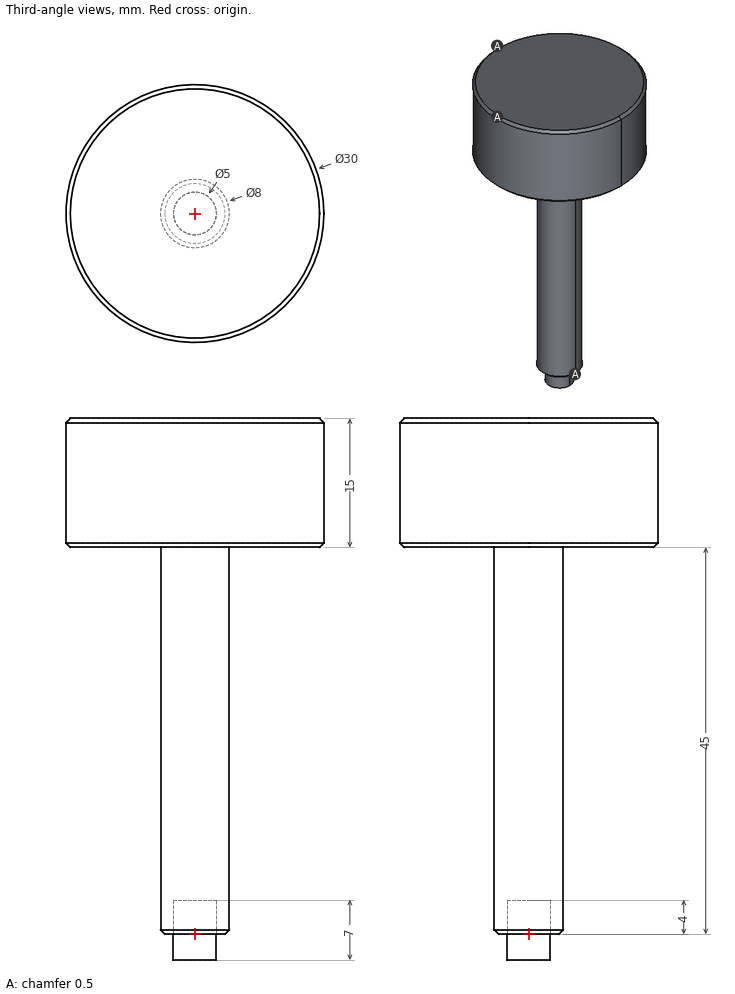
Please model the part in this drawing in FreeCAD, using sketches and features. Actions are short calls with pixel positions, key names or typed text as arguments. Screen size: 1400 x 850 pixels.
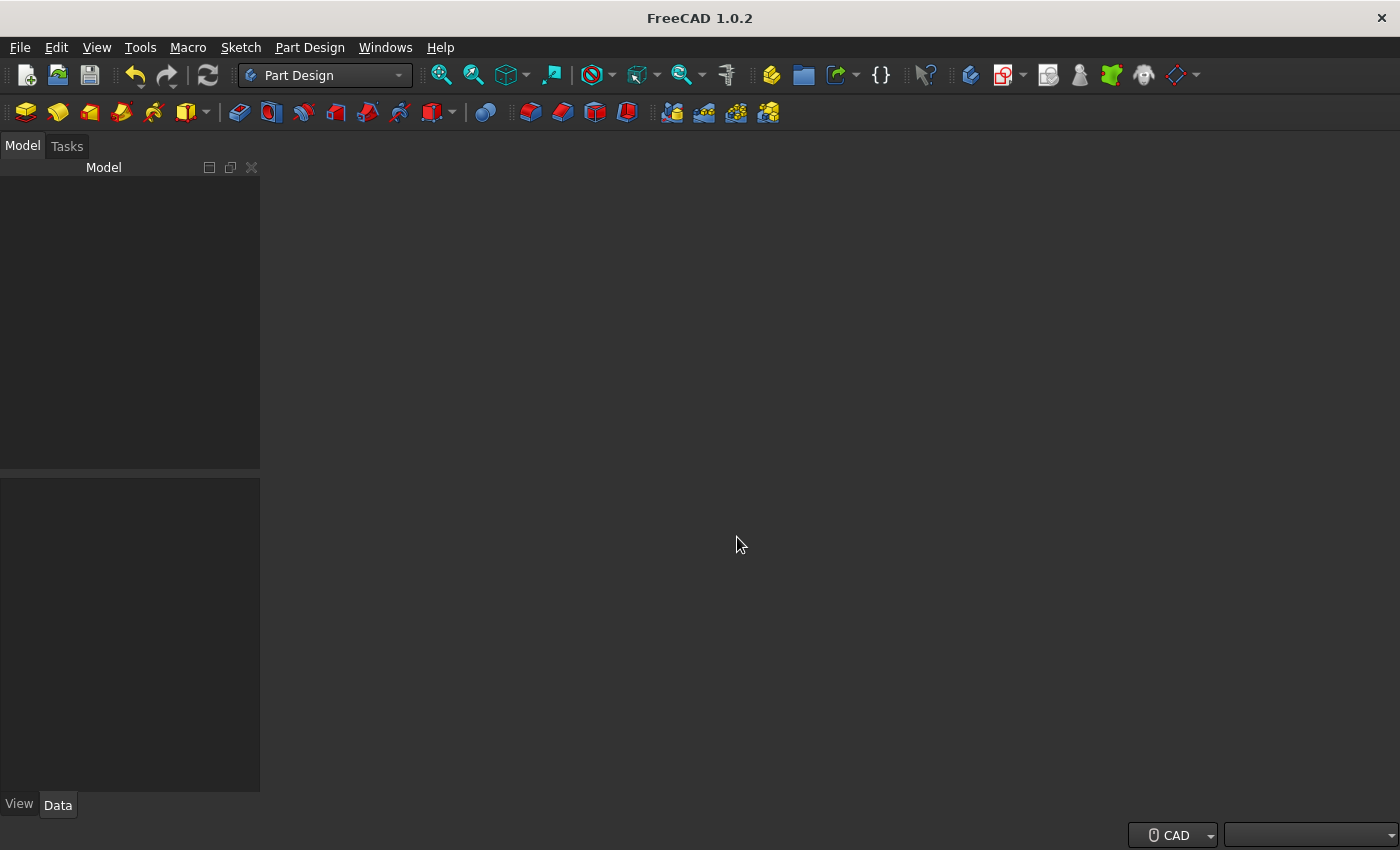
click(26, 76)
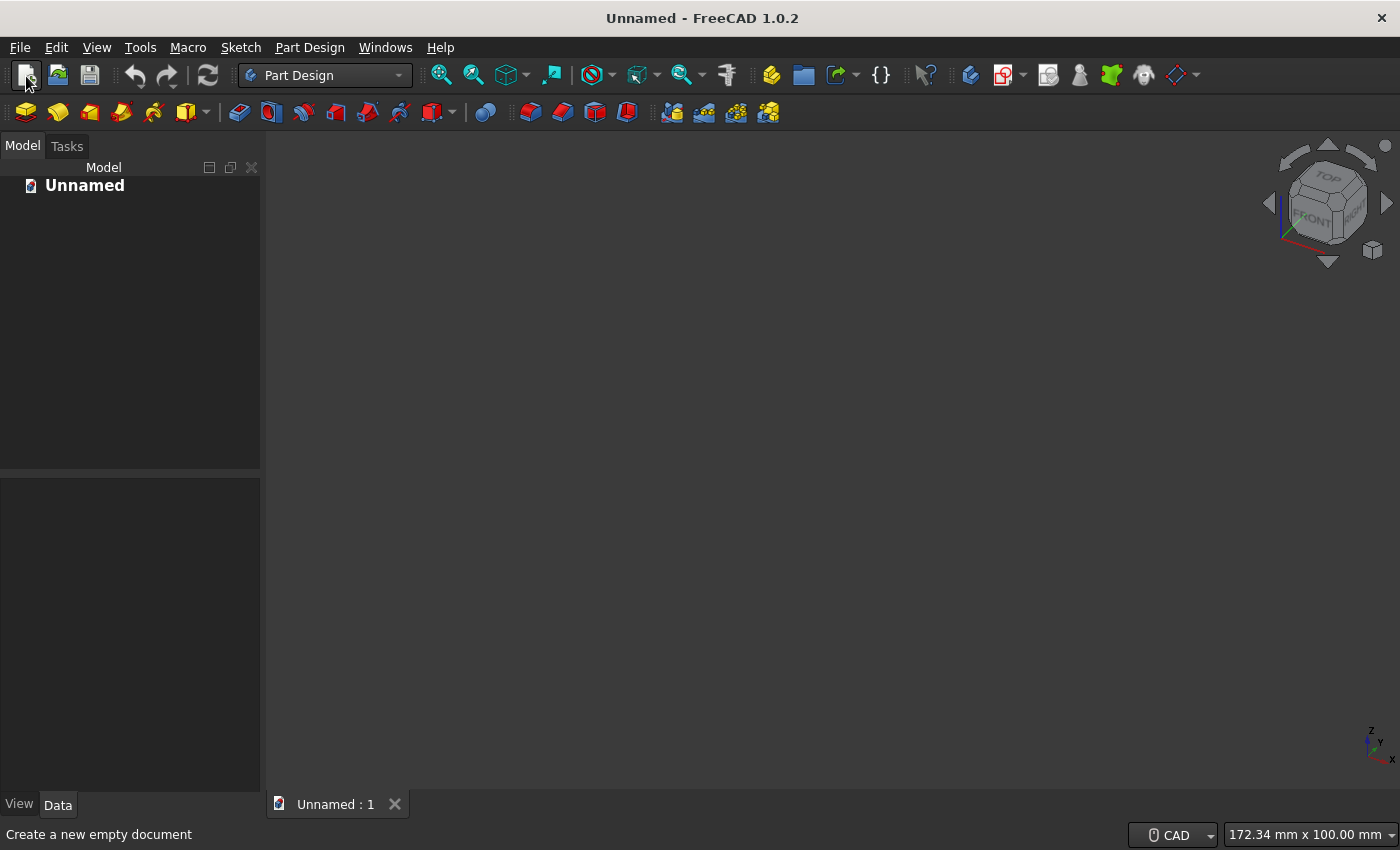
click(1004, 76)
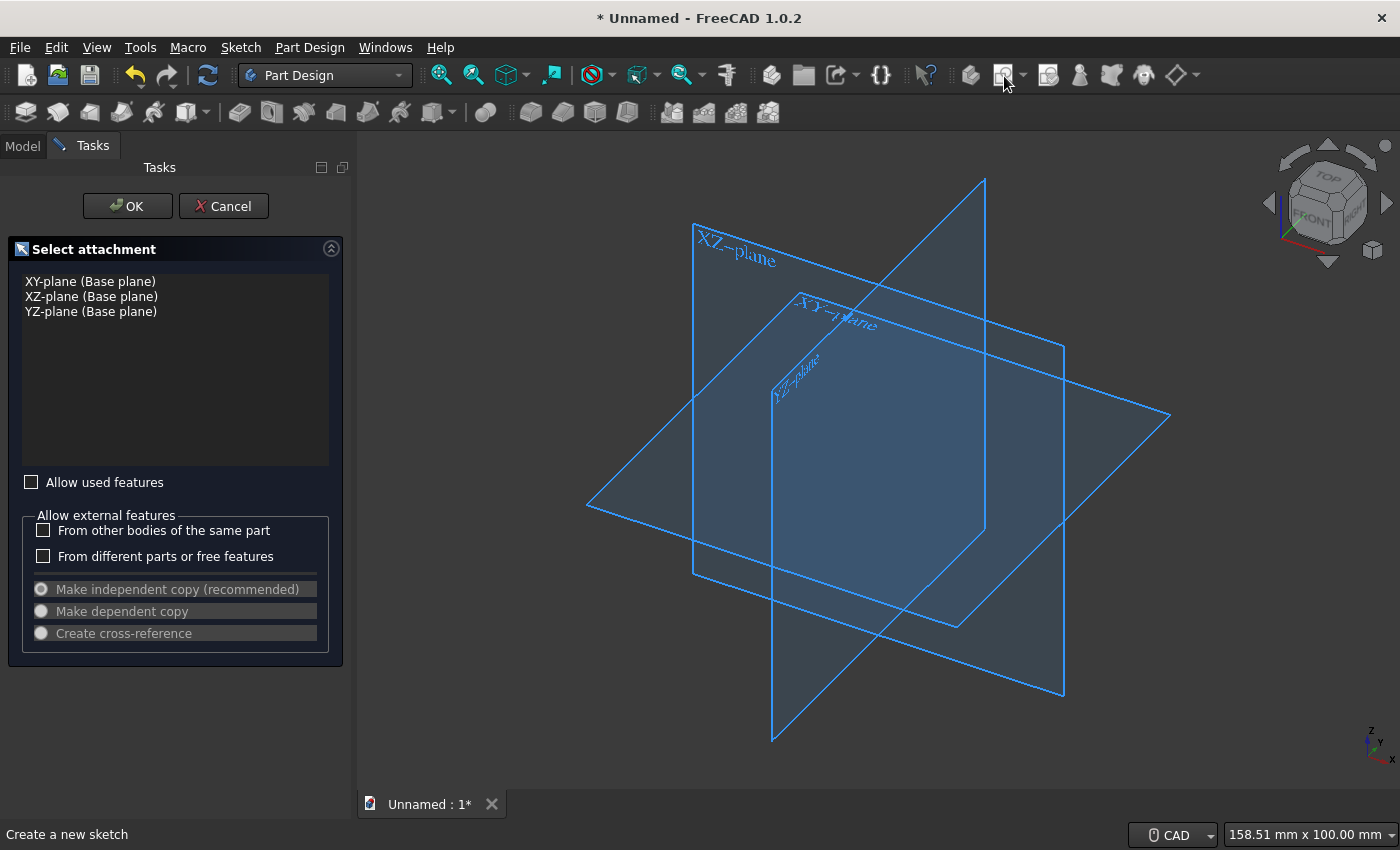
click(82, 282)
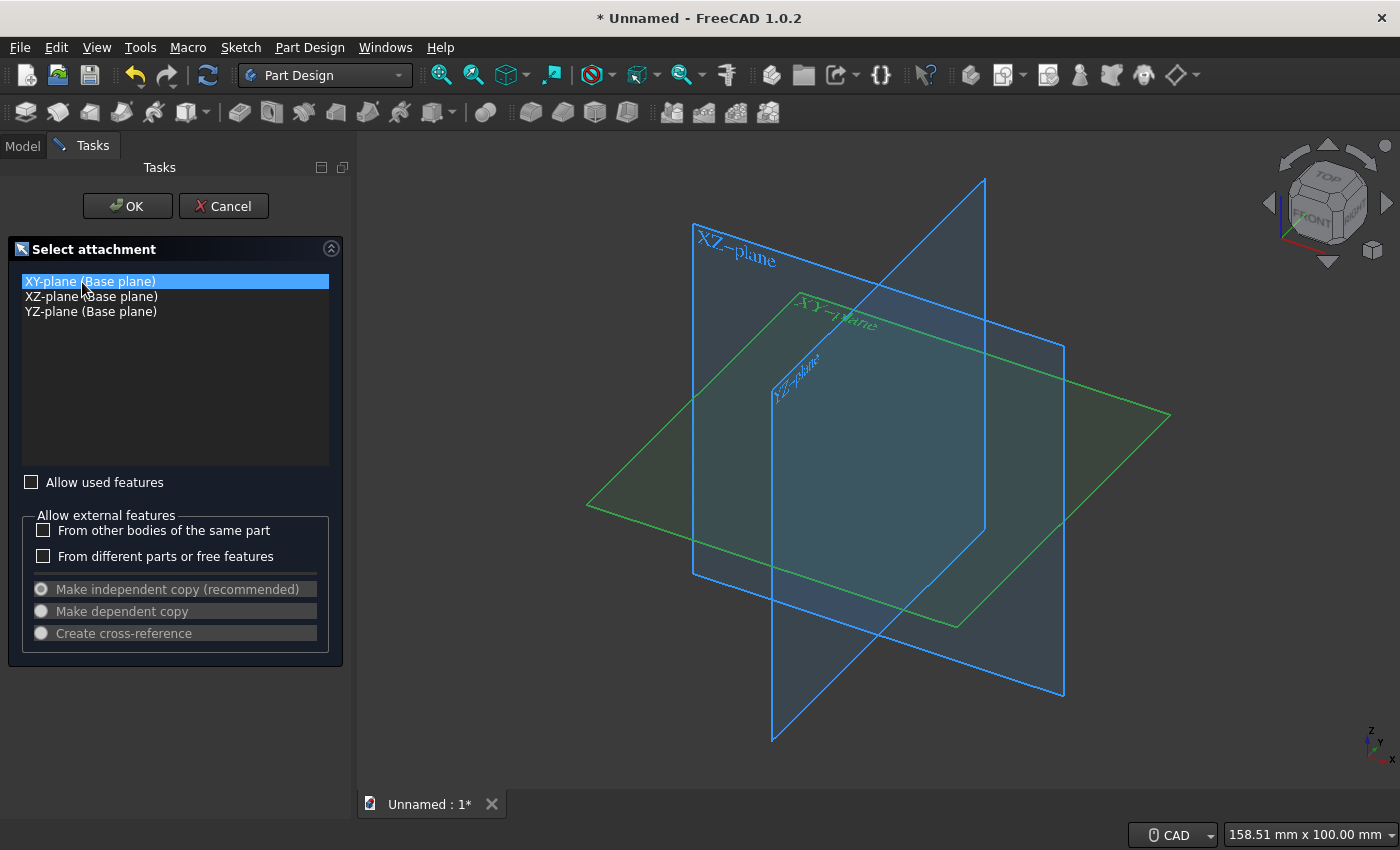
click(128, 206)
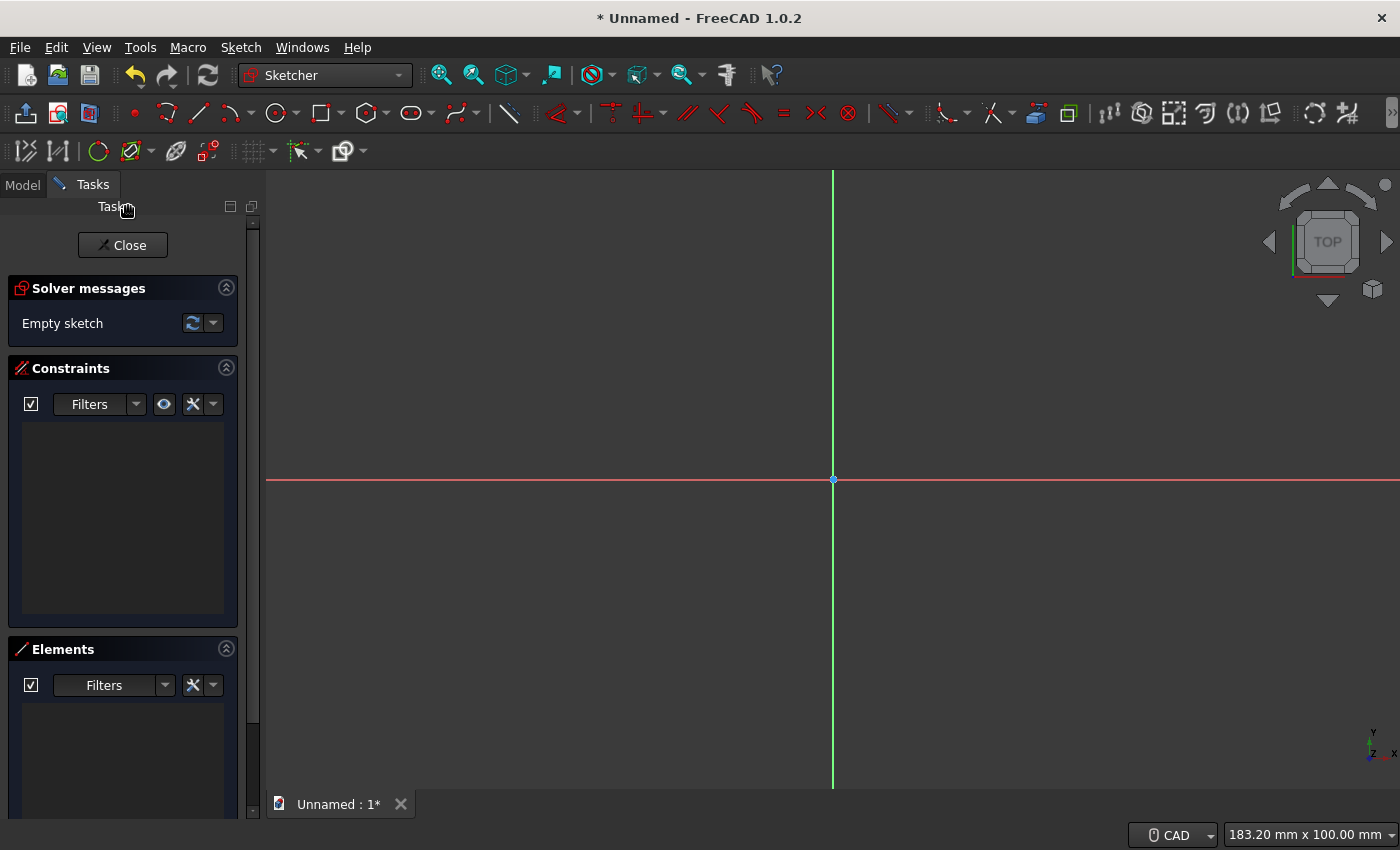
scroll(844, 480, up, 10)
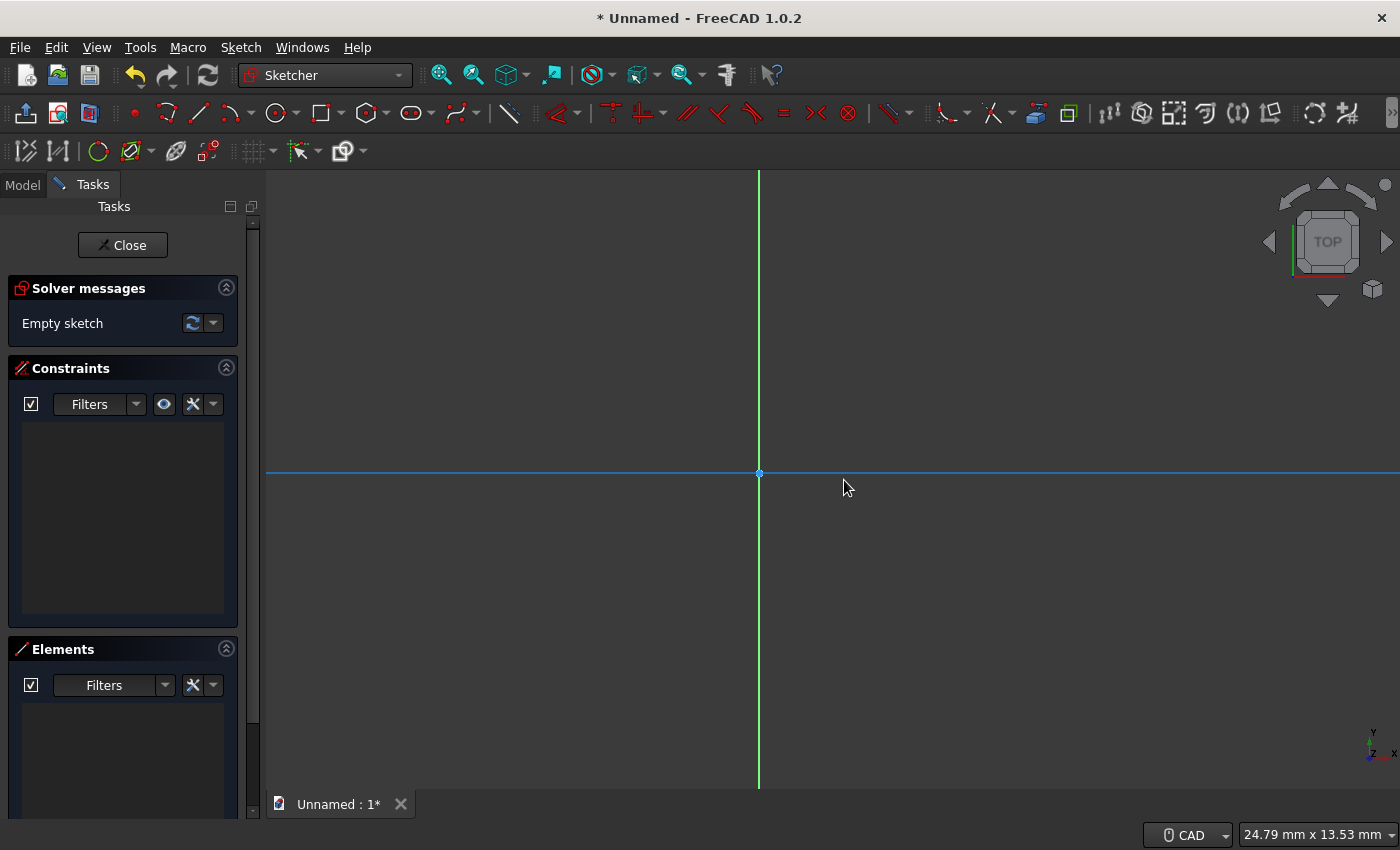
click(276, 114)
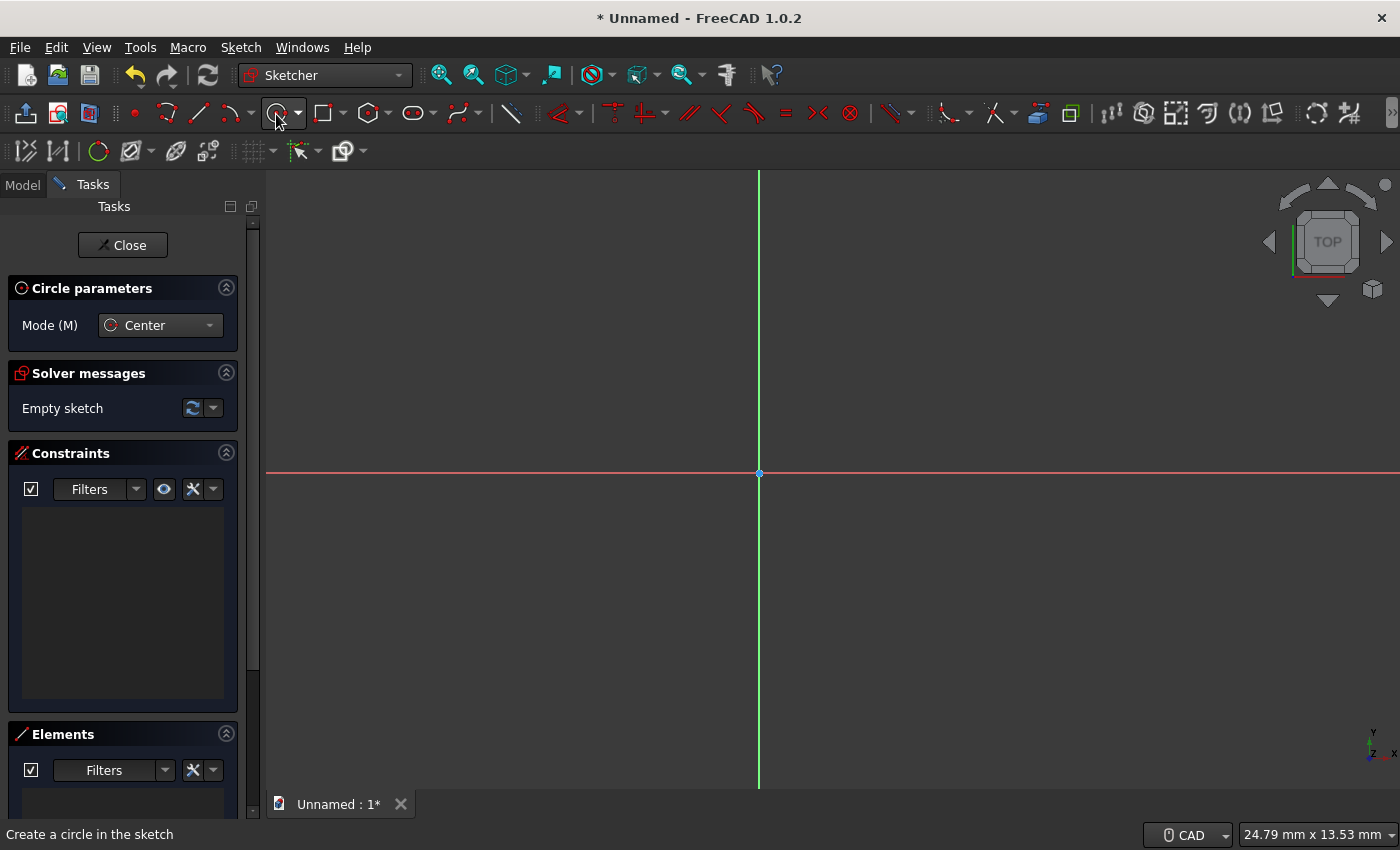
click(759, 473)
move(889, 344)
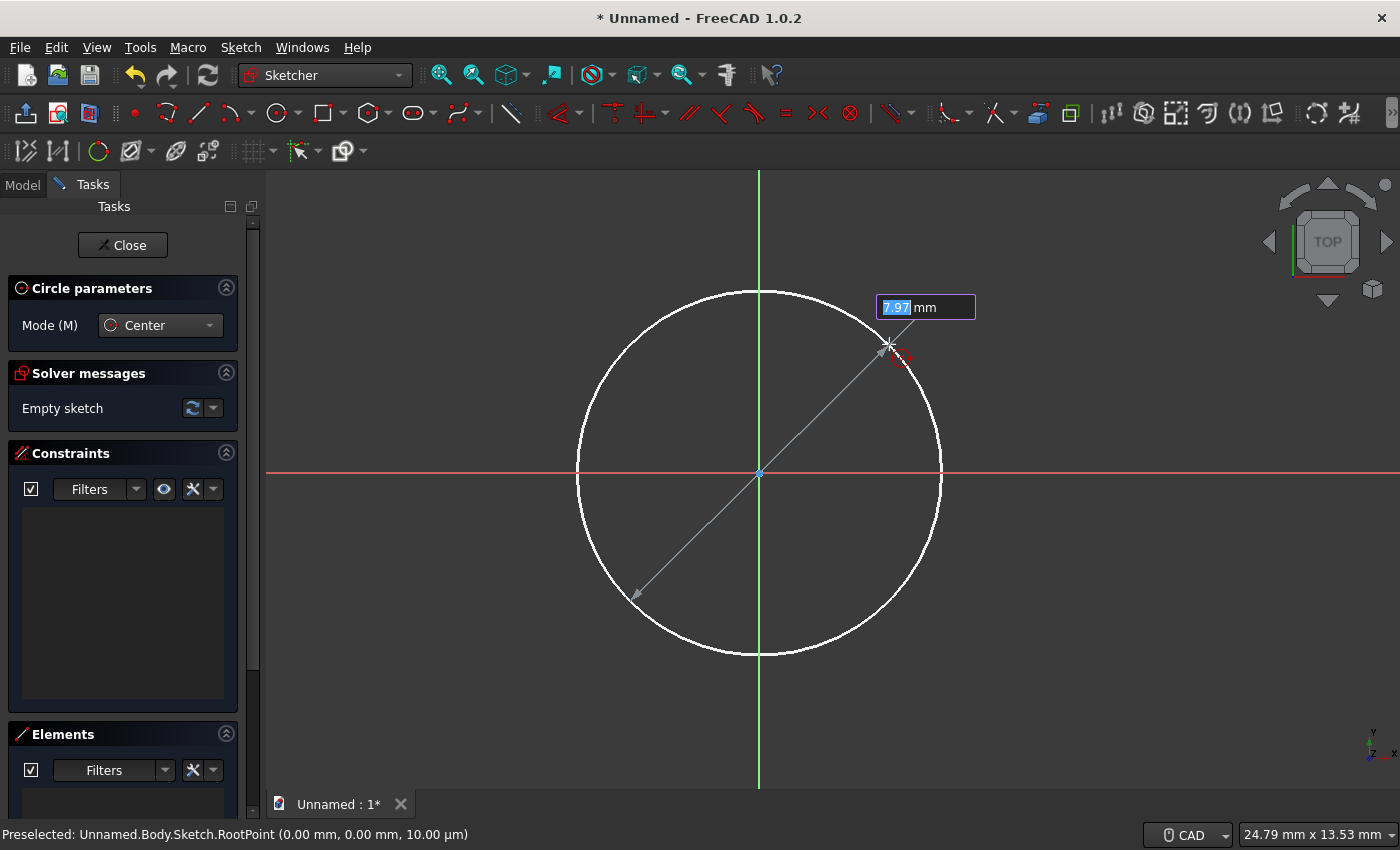
text(8)
key(Return)
key(Escape)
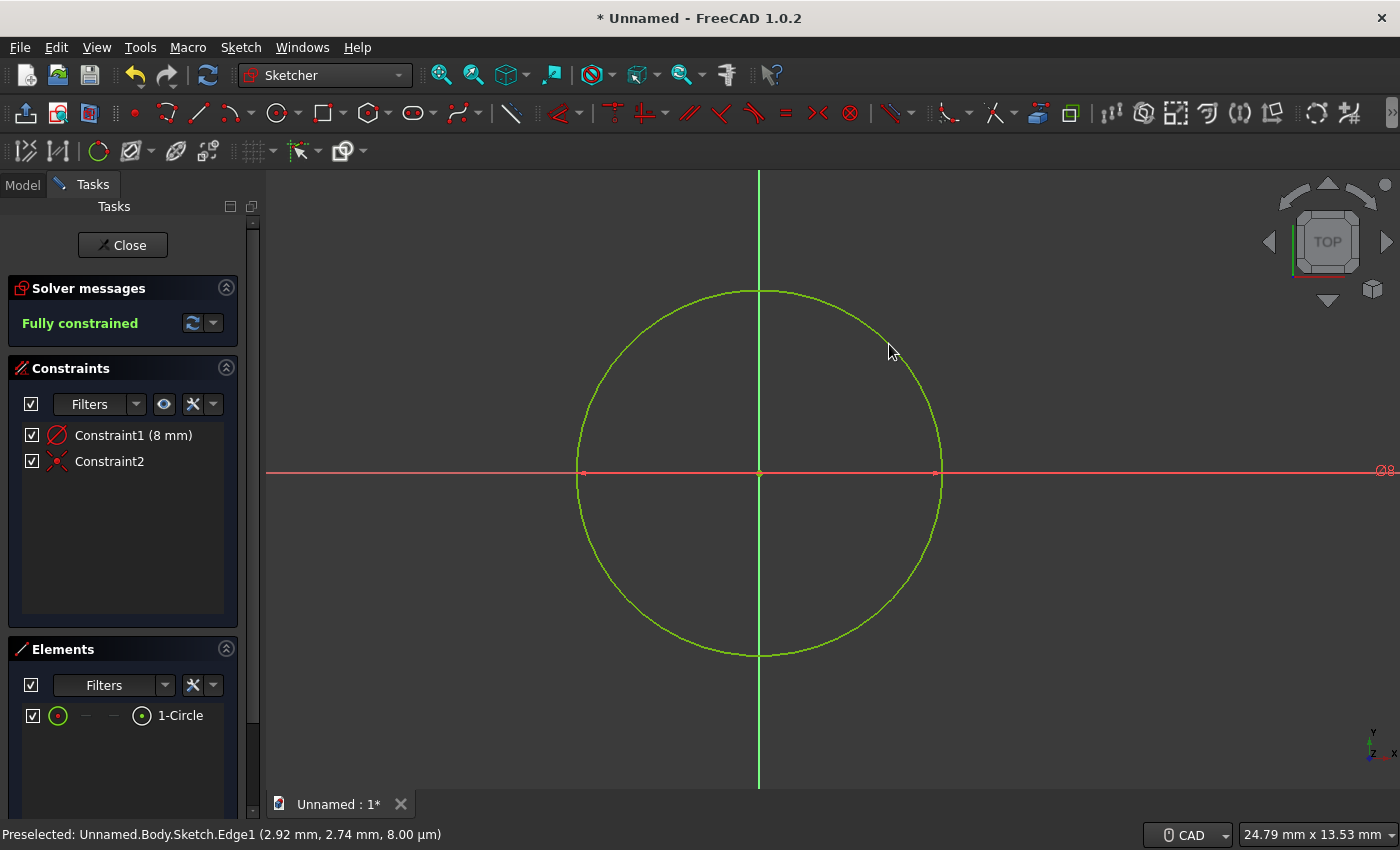
click(123, 245)